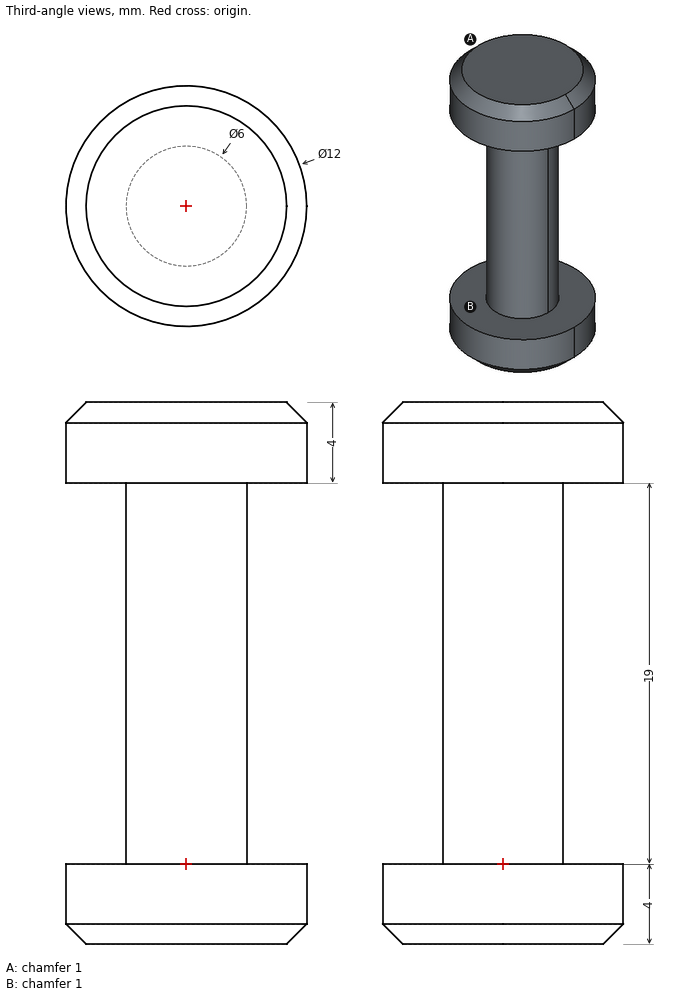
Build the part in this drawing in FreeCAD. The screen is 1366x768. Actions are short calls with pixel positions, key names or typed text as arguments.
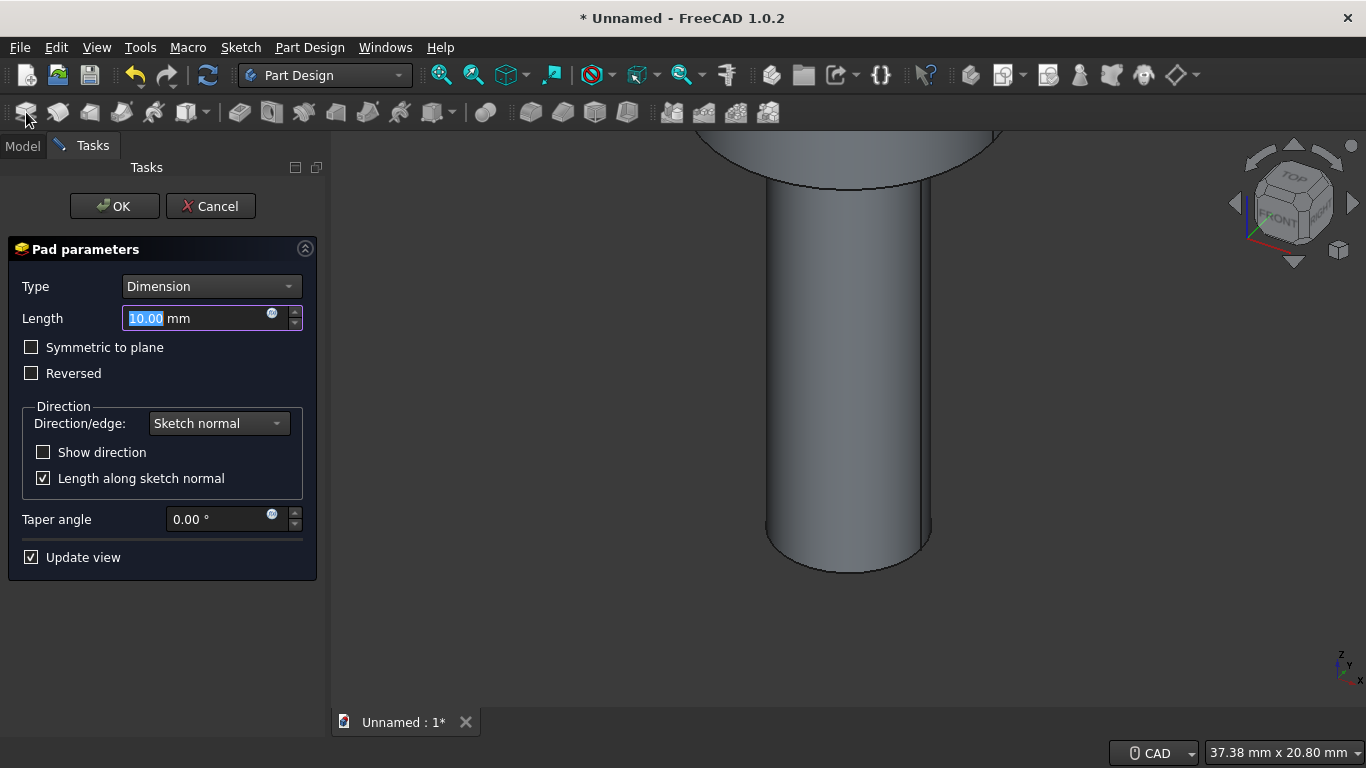
text(4)
key(Tab)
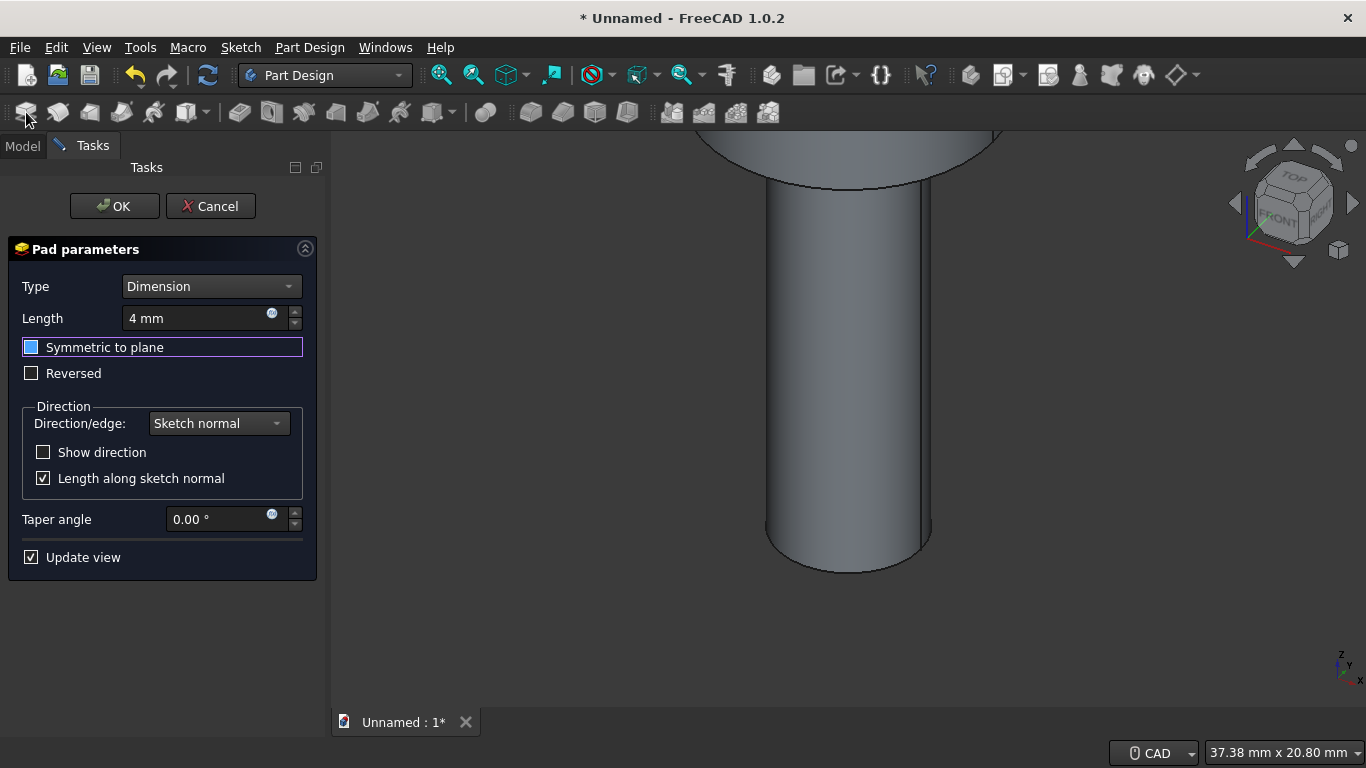
click(115, 206)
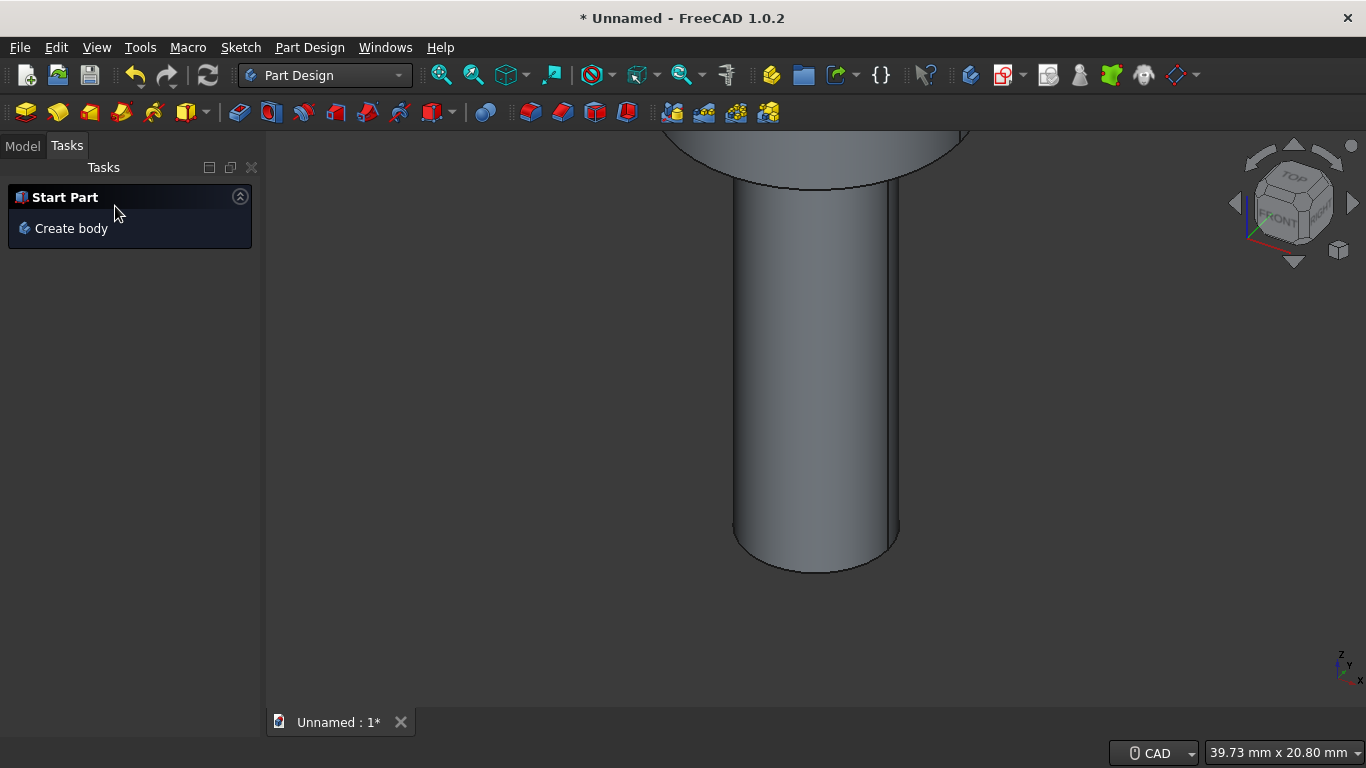
key(v)
key(f)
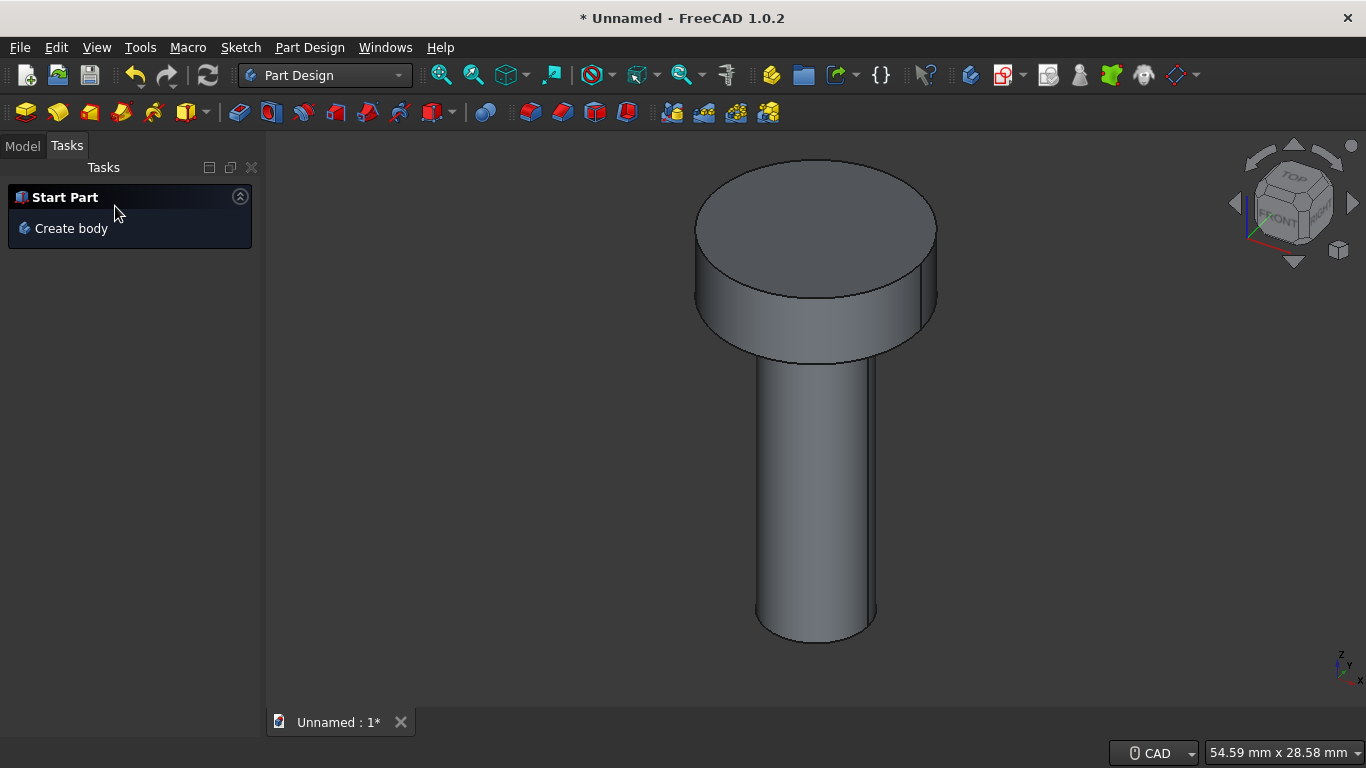
click(696, 235)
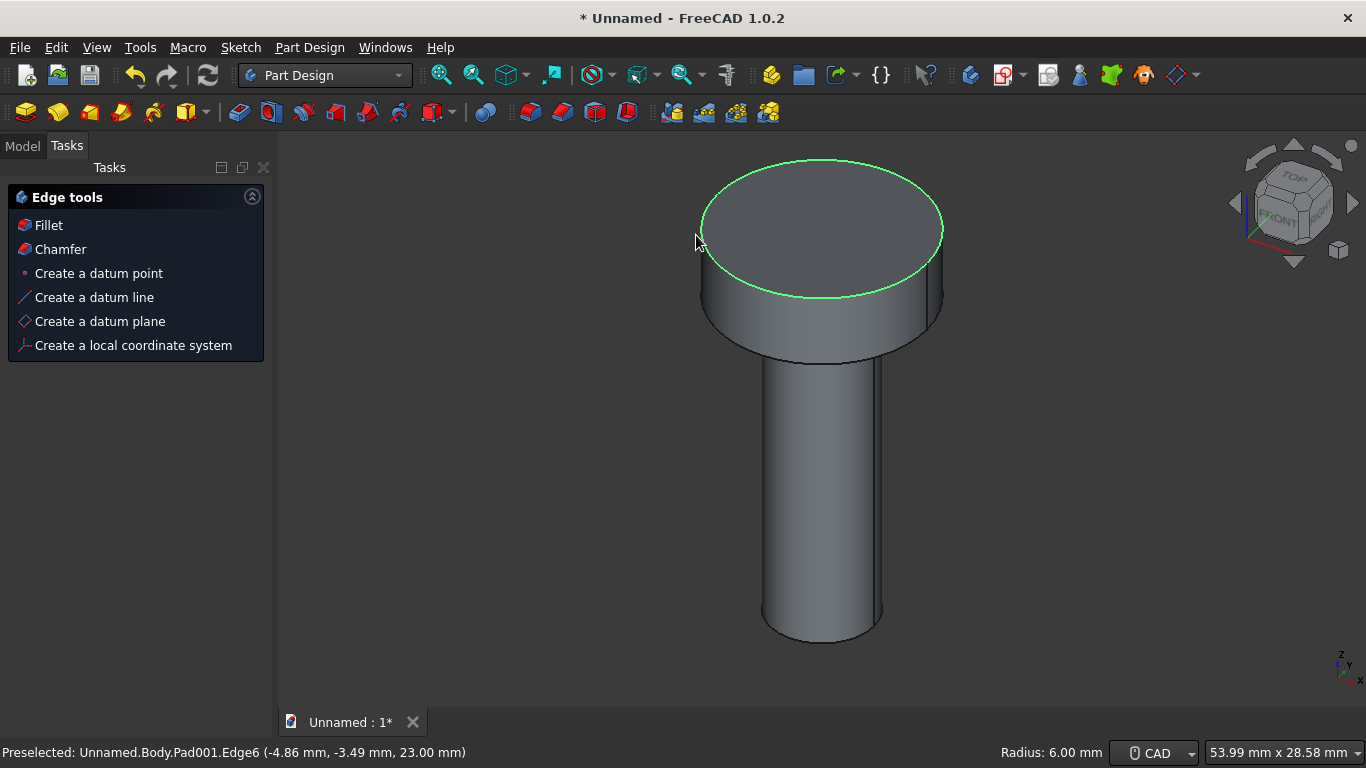
click(564, 112)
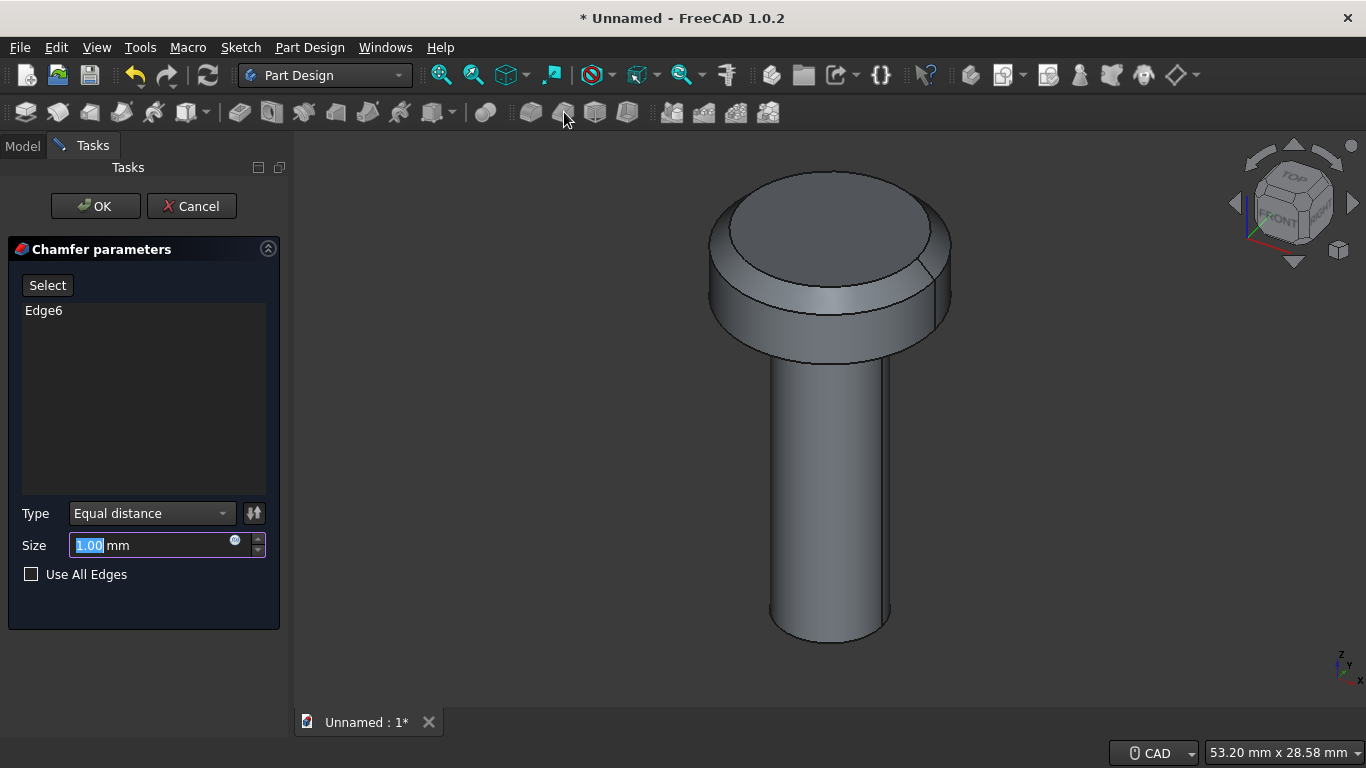
text(1)
key(Tab)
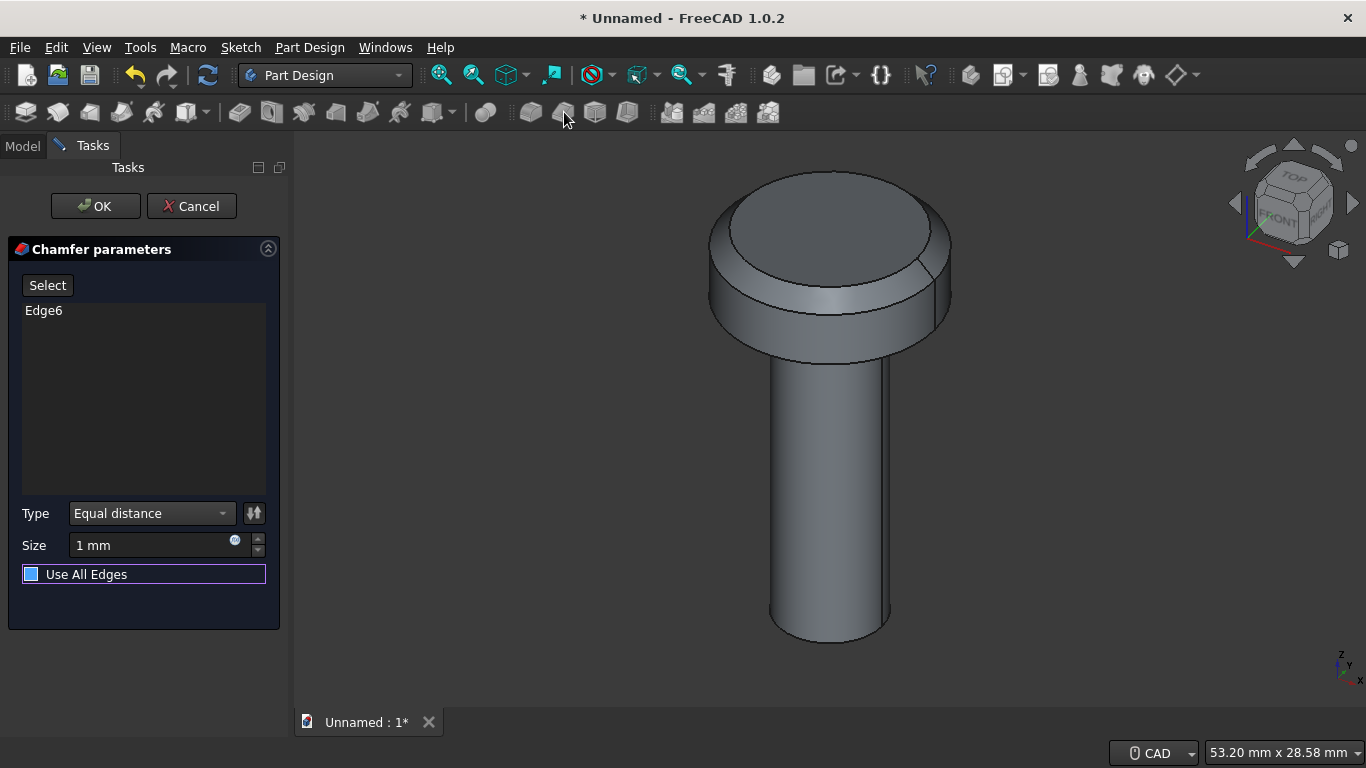
click(96, 206)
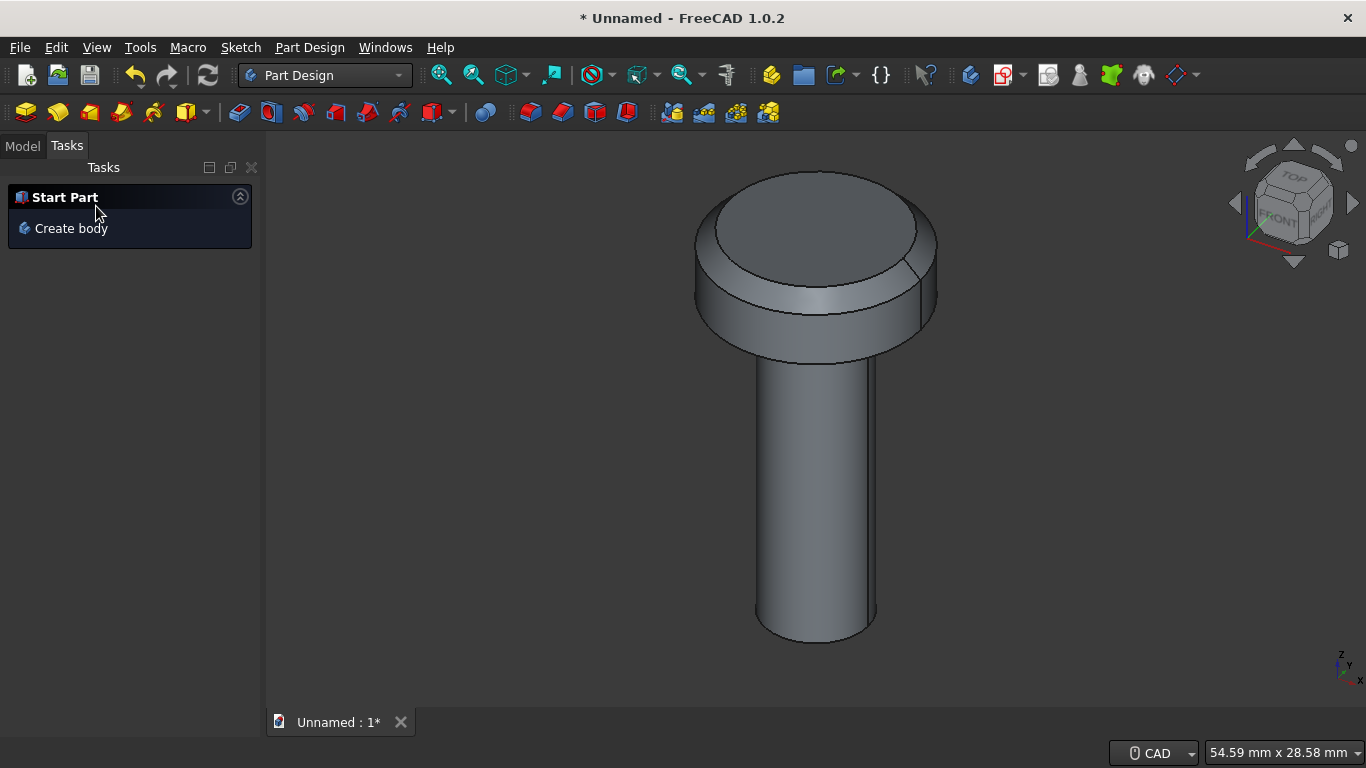
click(23, 145)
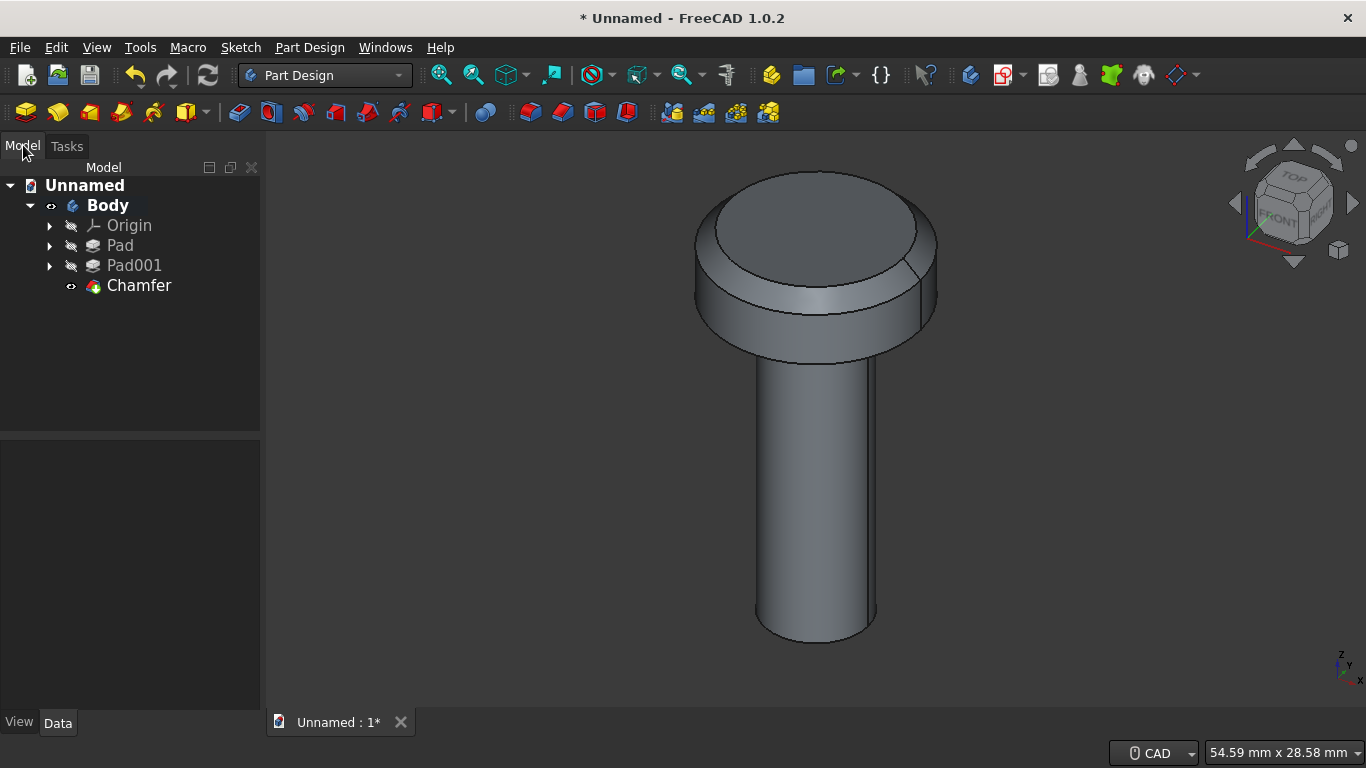
click(50, 226)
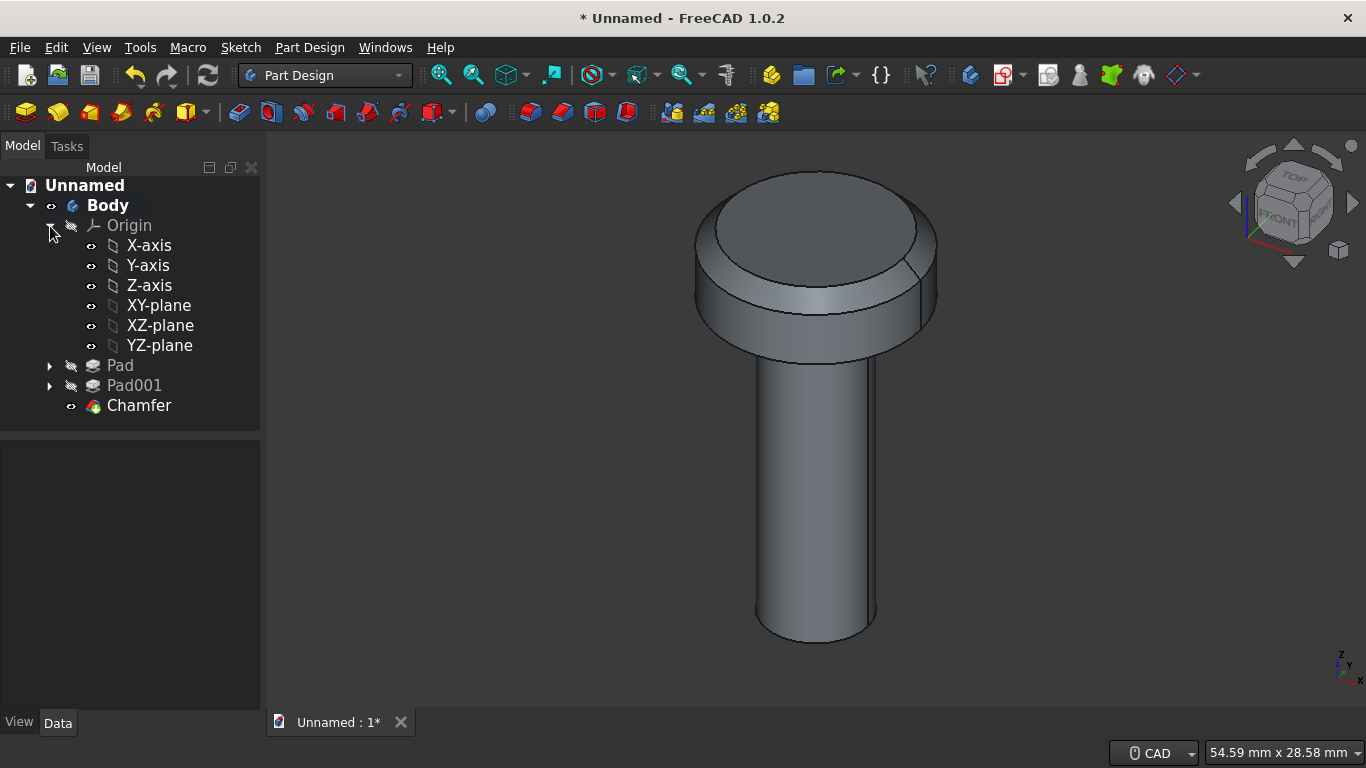
click(136, 306)